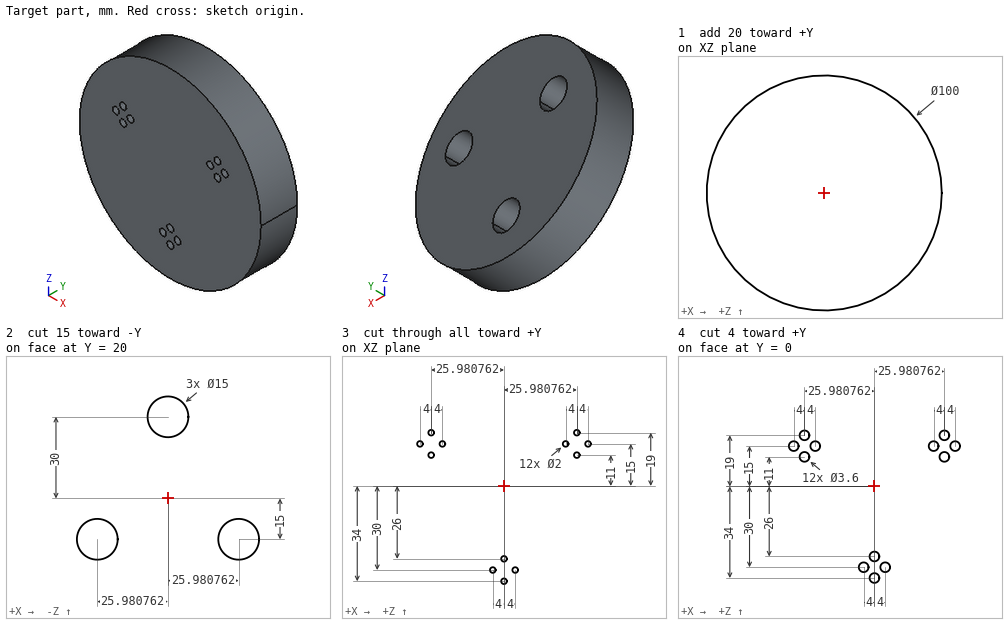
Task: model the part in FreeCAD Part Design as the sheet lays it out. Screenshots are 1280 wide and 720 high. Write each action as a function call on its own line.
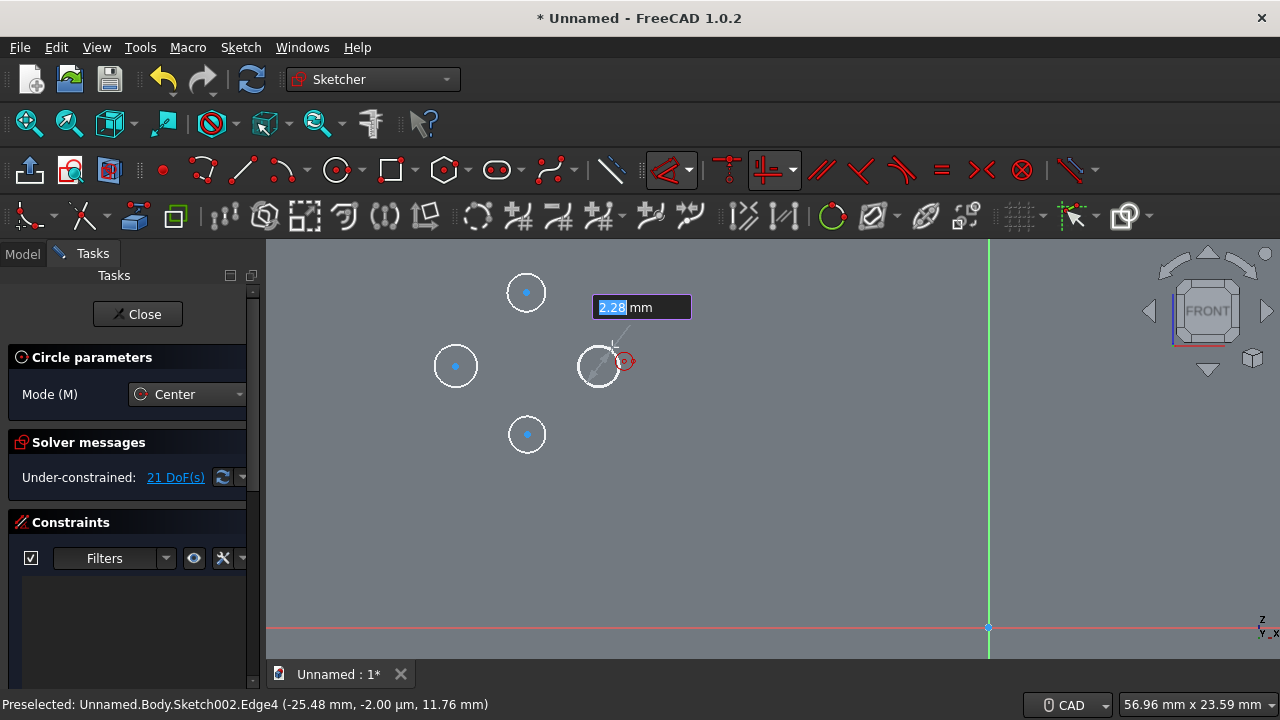
click(610, 348)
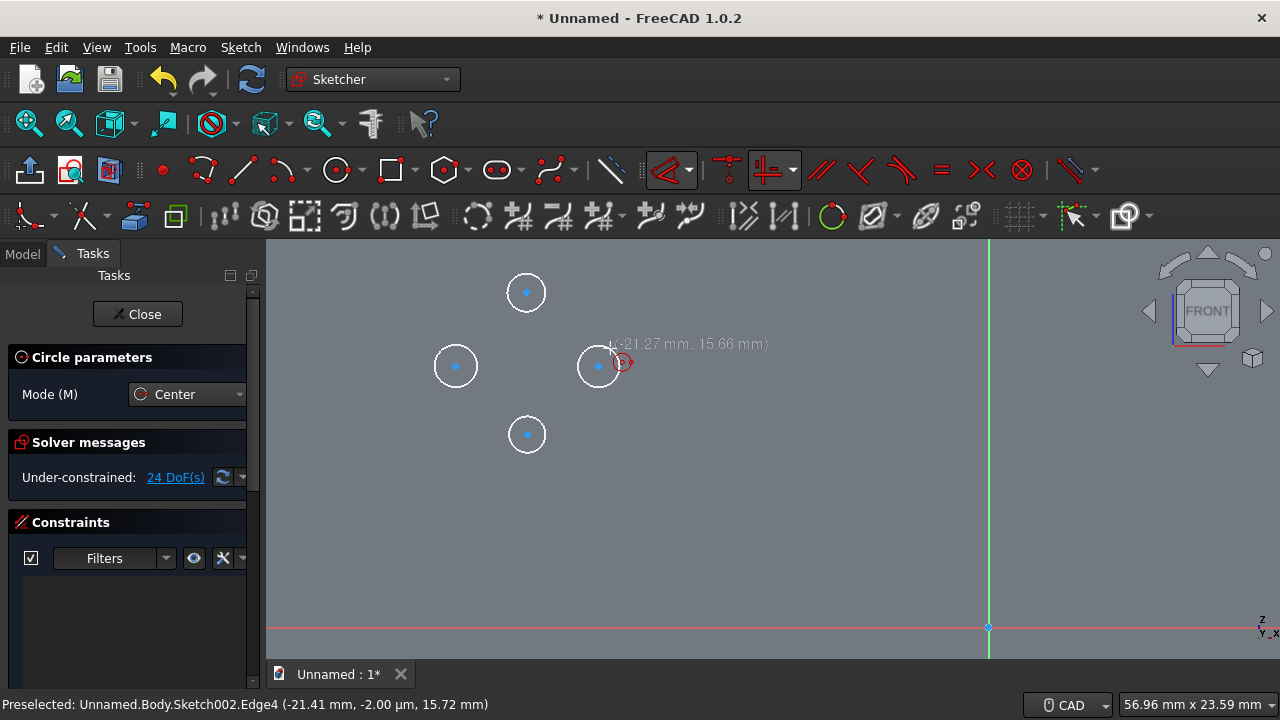
scroll(611, 347, down, 7)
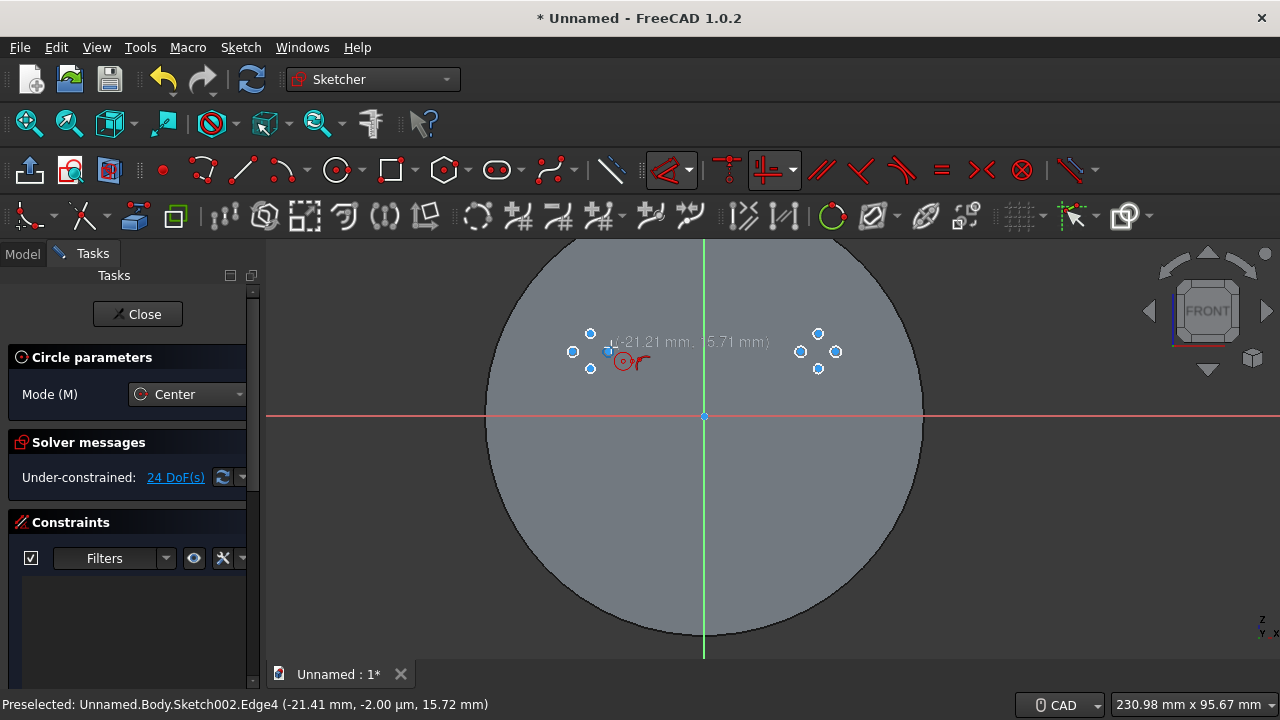
scroll(704, 531, up, 9)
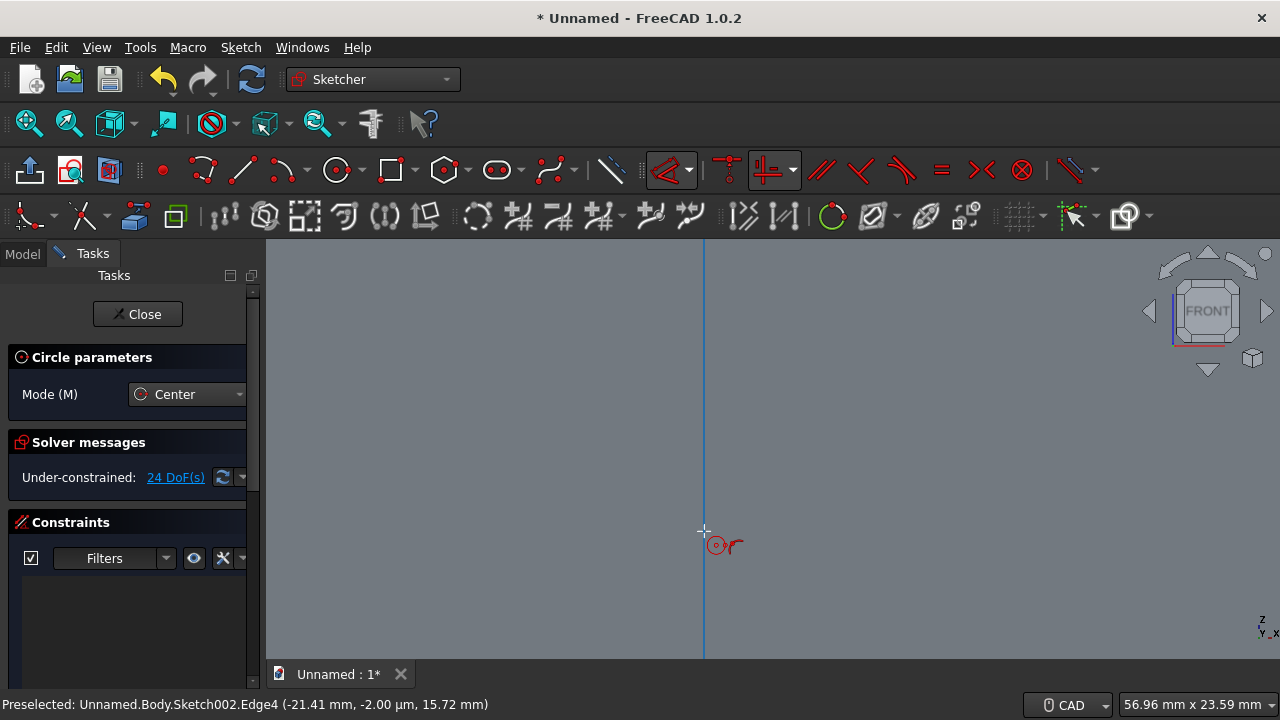
scroll(705, 531, down, 9)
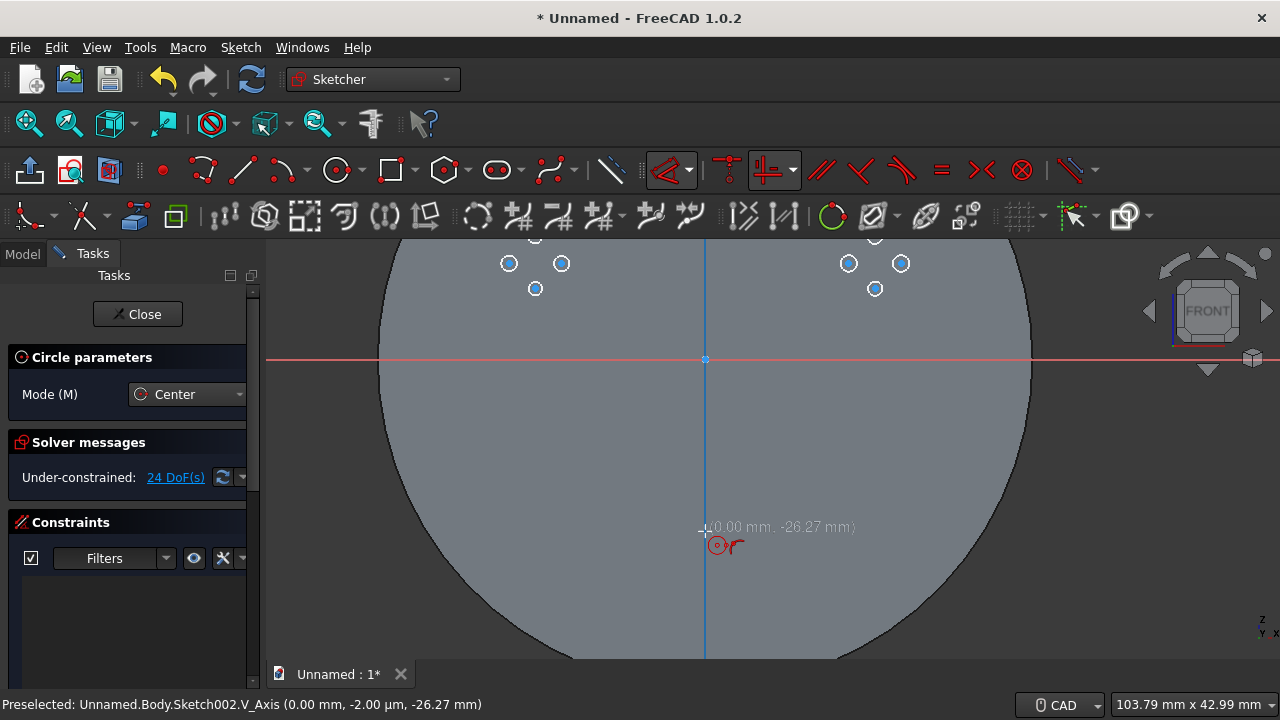
click(705, 531)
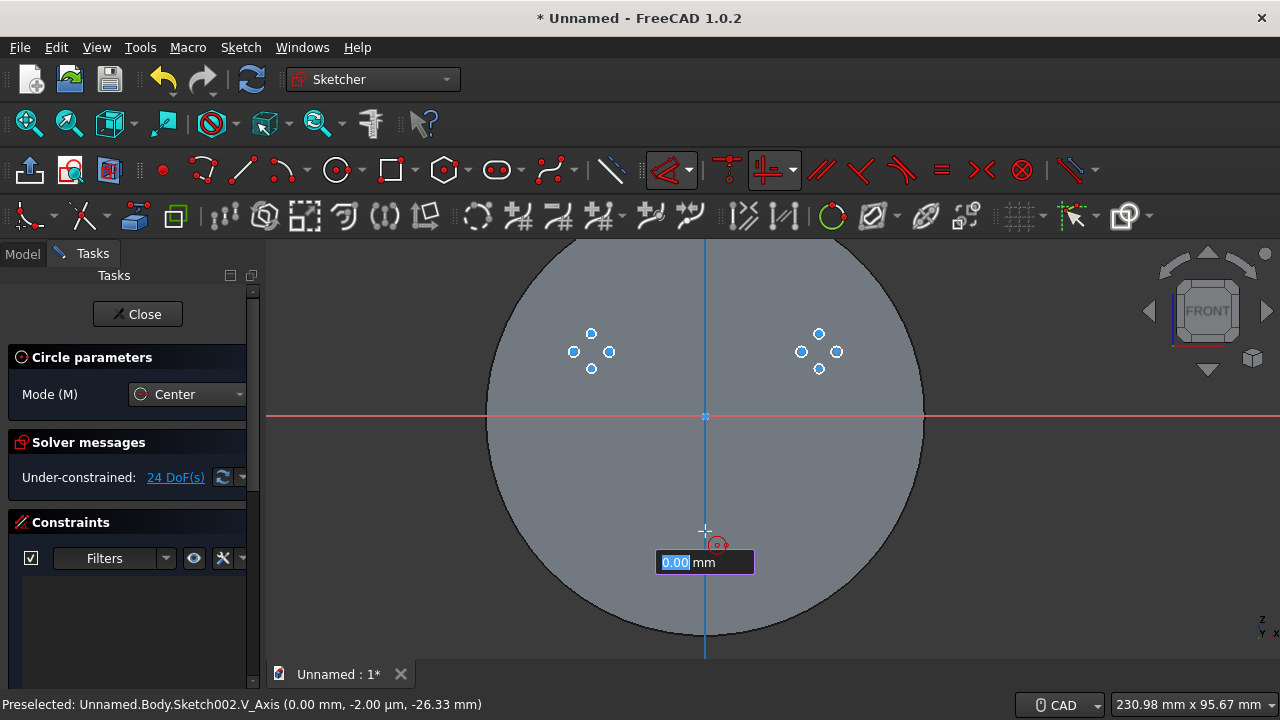
scroll(709, 529, up, 7)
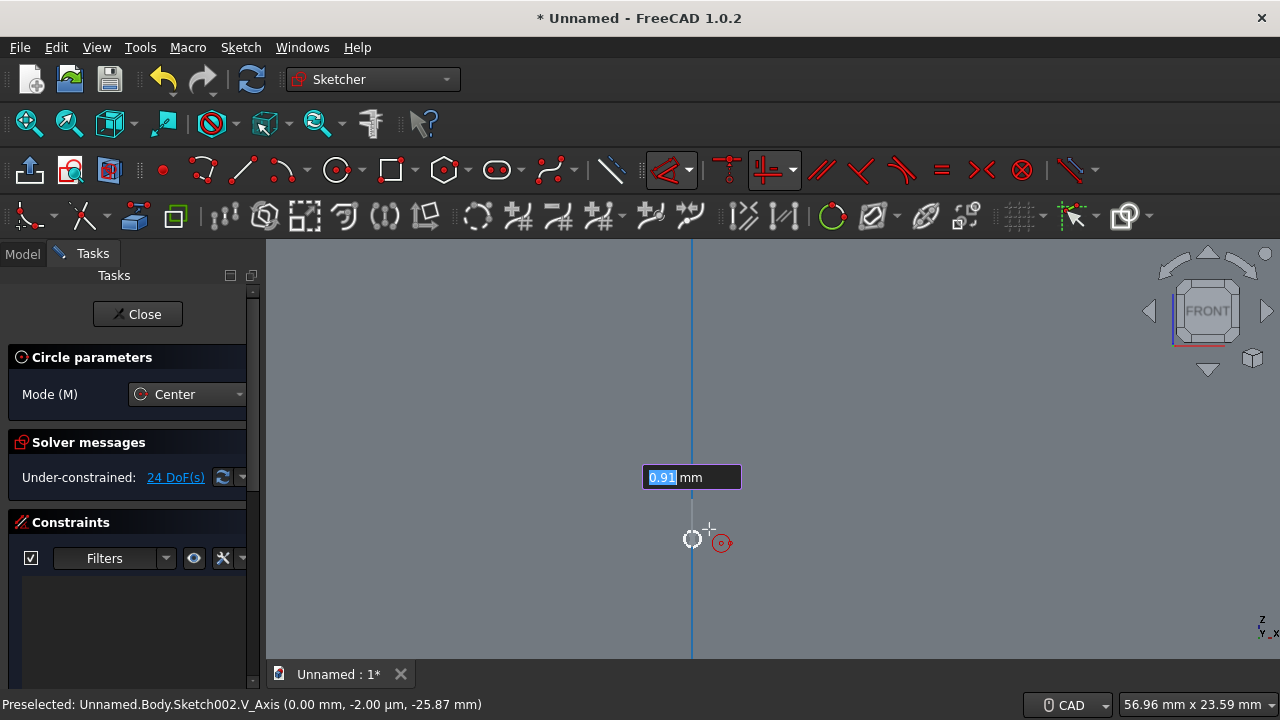
click(709, 527)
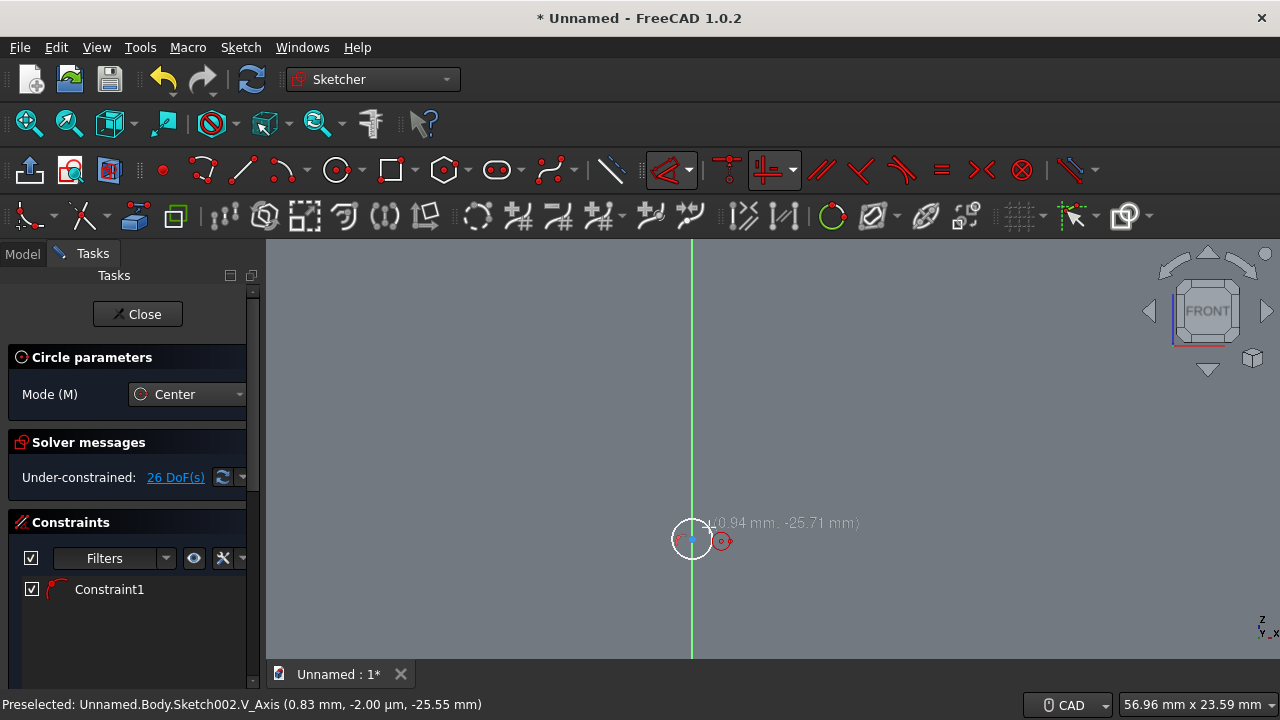
scroll(621, 604, up, 2)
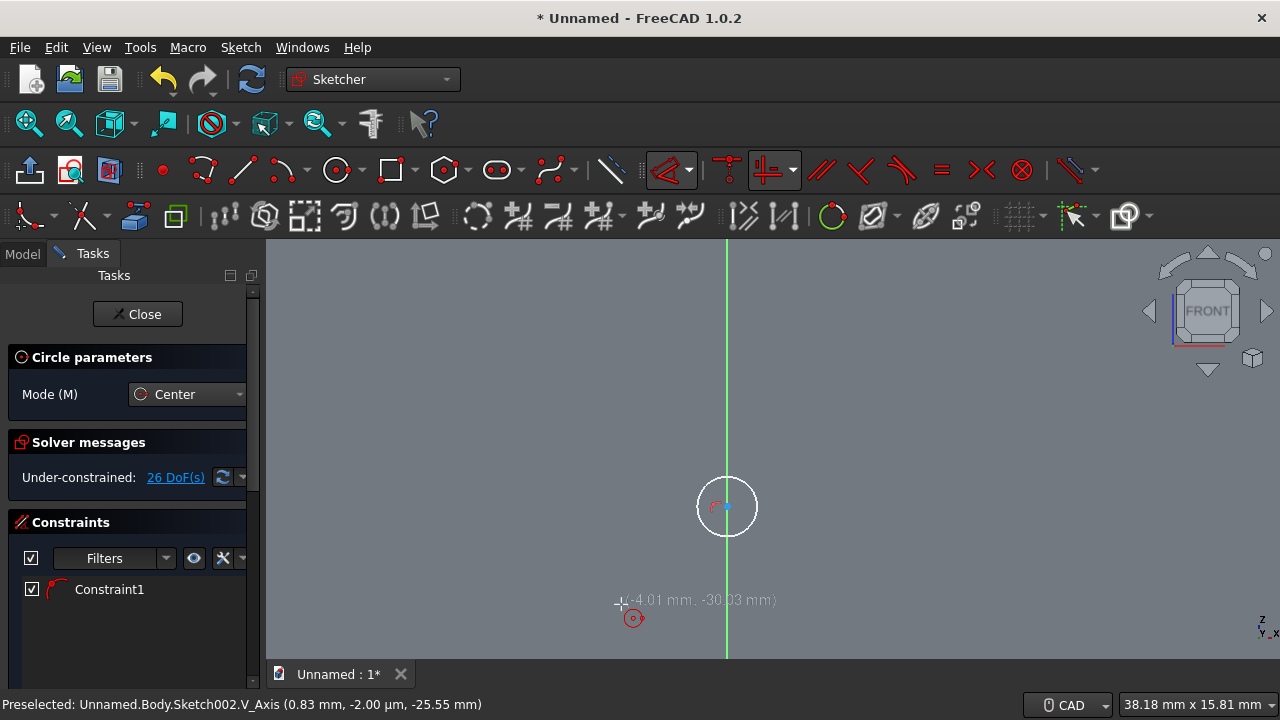
scroll(700, 537, down, 9)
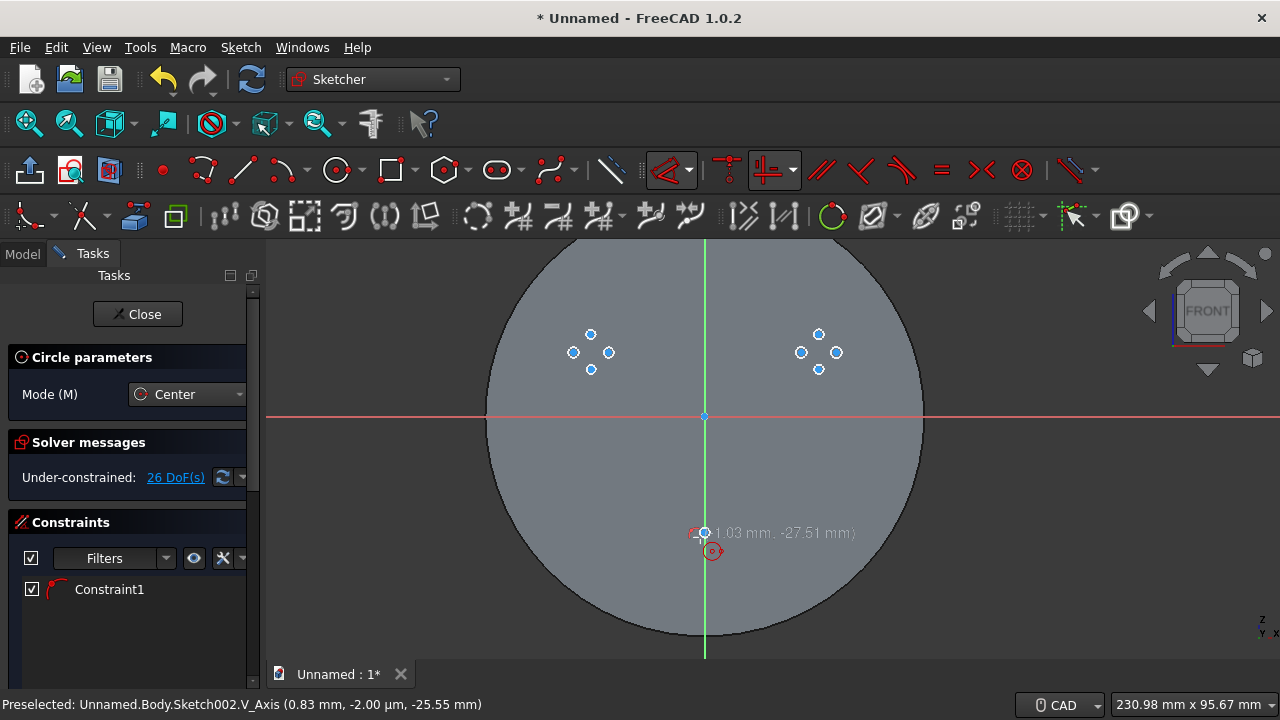
click(687, 549)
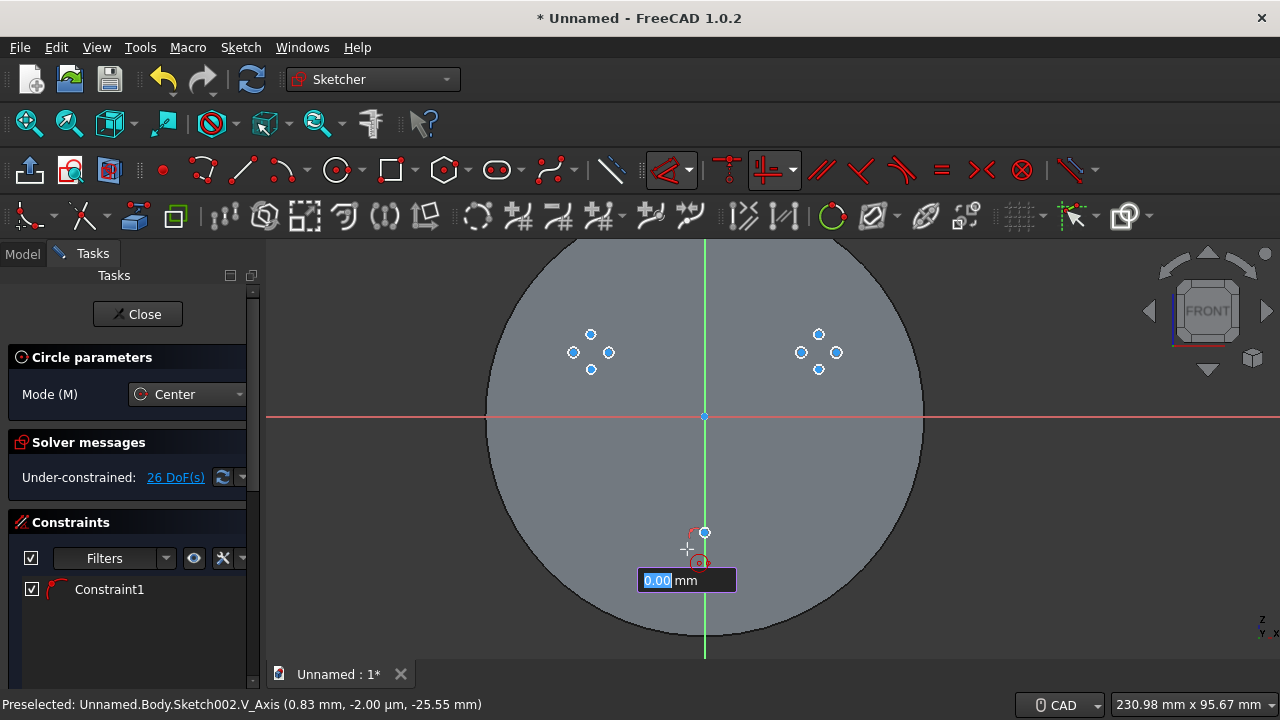
scroll(690, 546, up, 7)